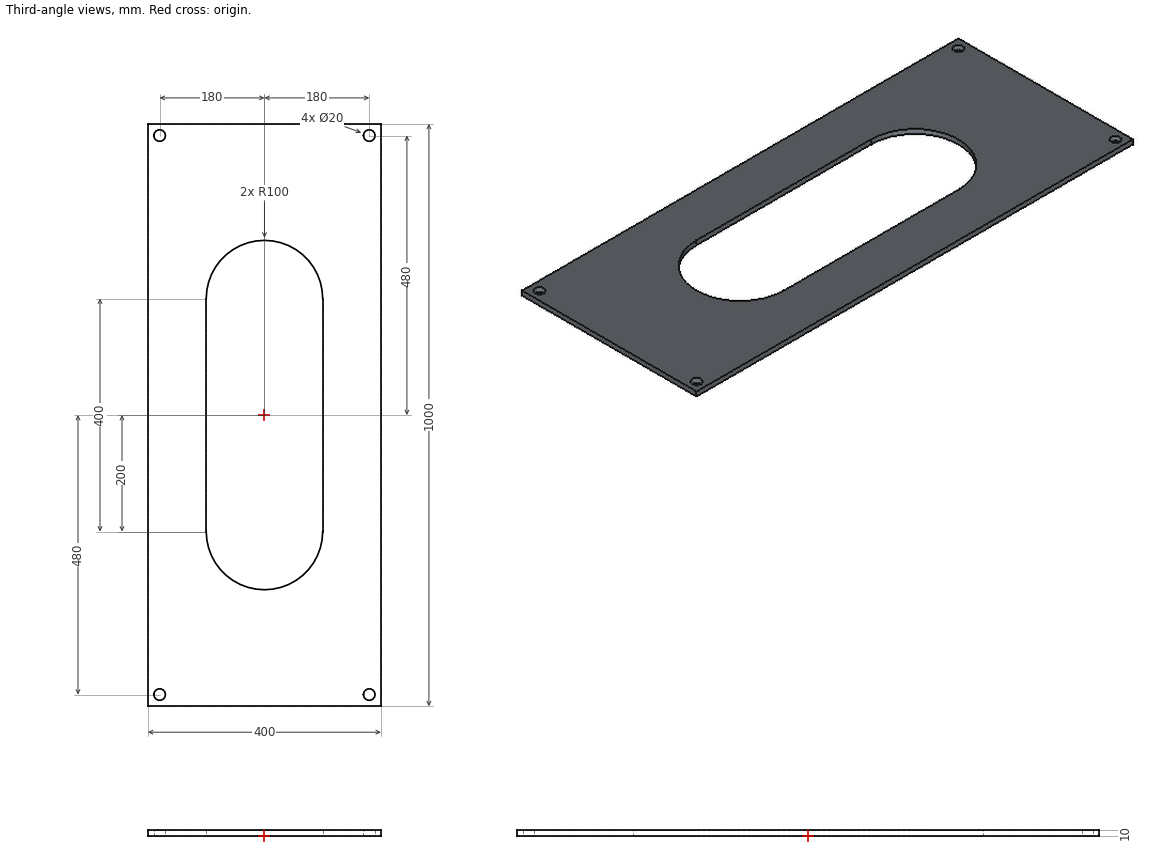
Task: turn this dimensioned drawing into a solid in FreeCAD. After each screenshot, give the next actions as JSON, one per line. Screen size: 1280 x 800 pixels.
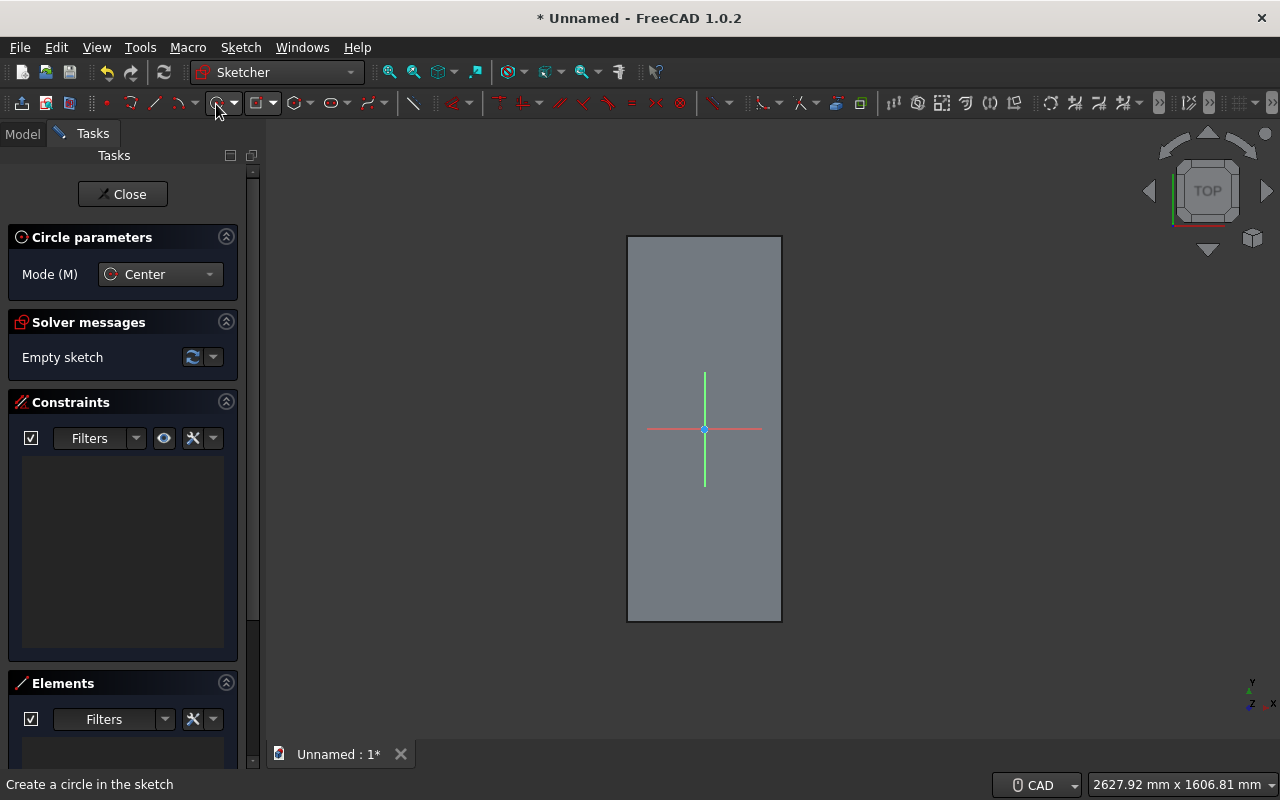
{"action": "scroll", "coordinate": [774, 244], "scroll_direction": "up", "scroll_amount": 9}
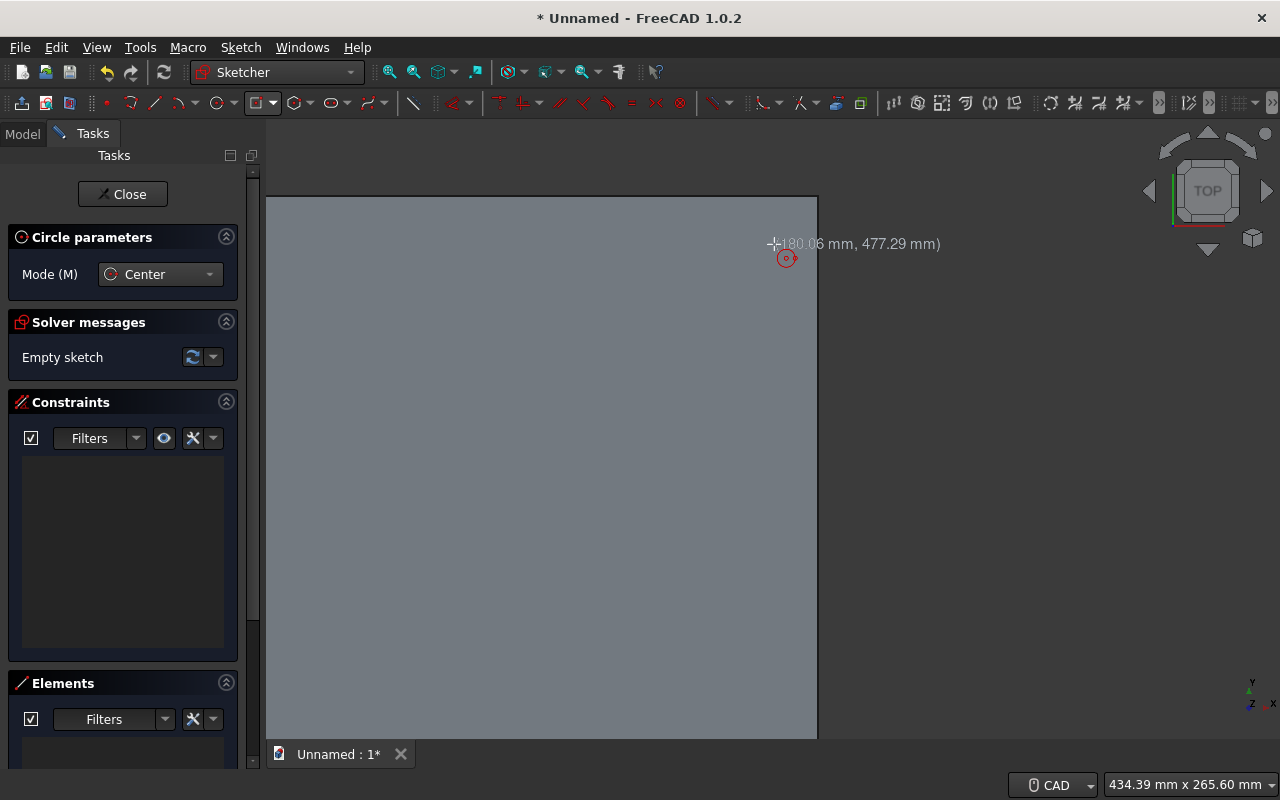
{"action": "scroll", "coordinate": [774, 244], "scroll_direction": "down", "scroll_amount": 9}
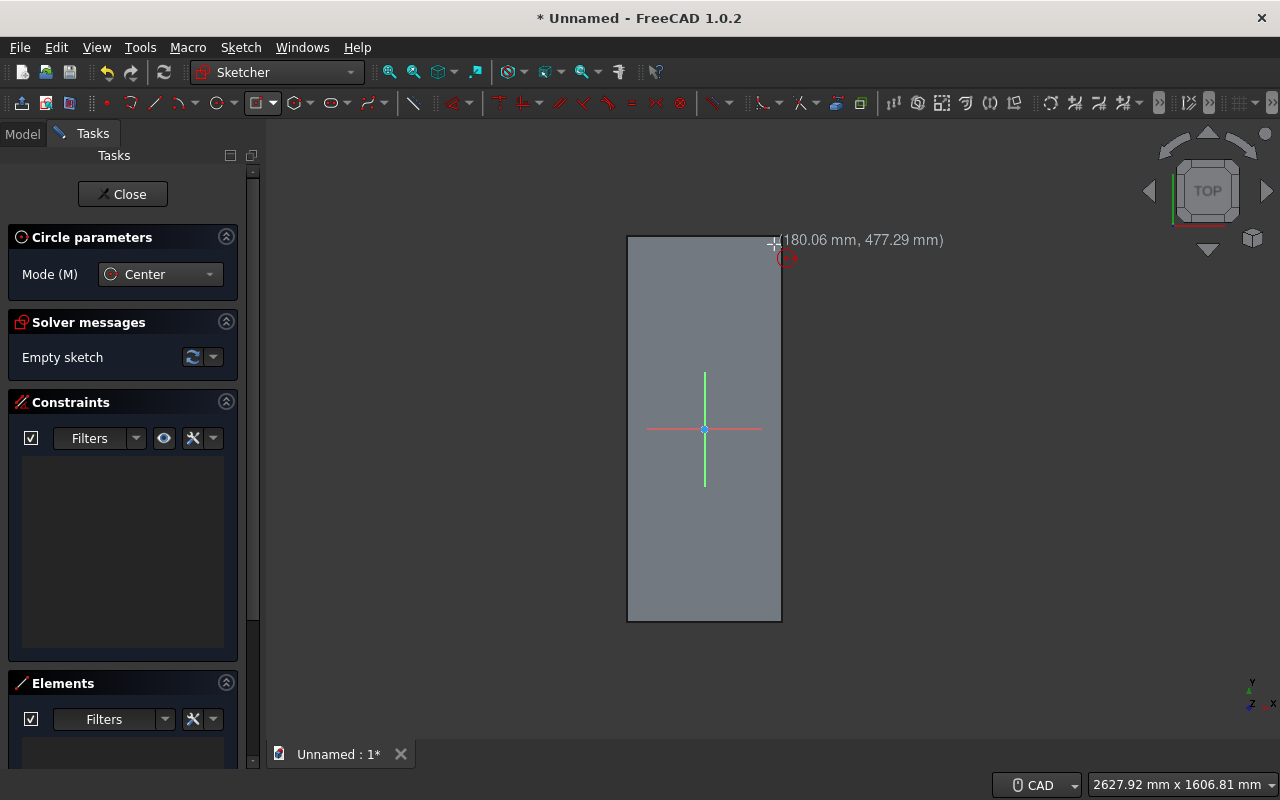
{"action": "left_click", "coordinate": [774, 244]}
{"action": "mouse_move", "coordinate": [777, 241]}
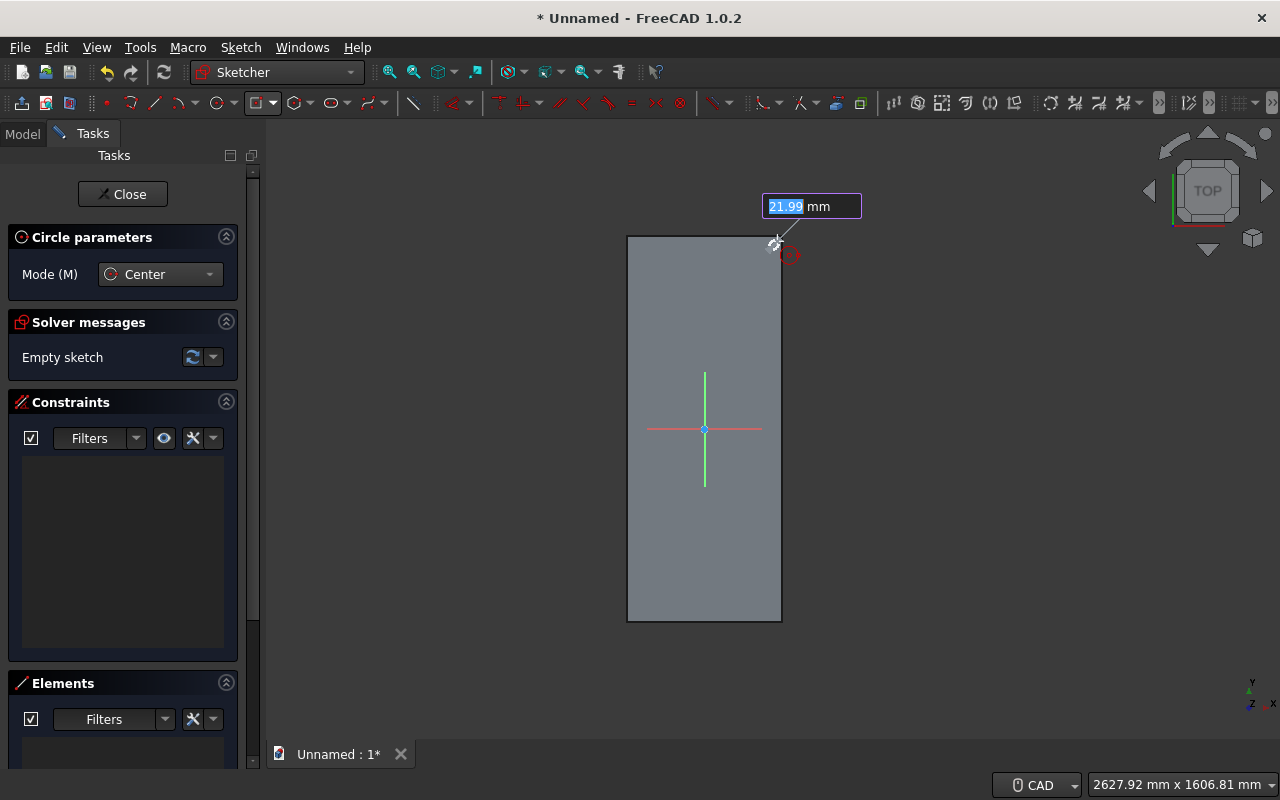
{"action": "type", "text": "20"}
{"action": "key", "text": "Return"}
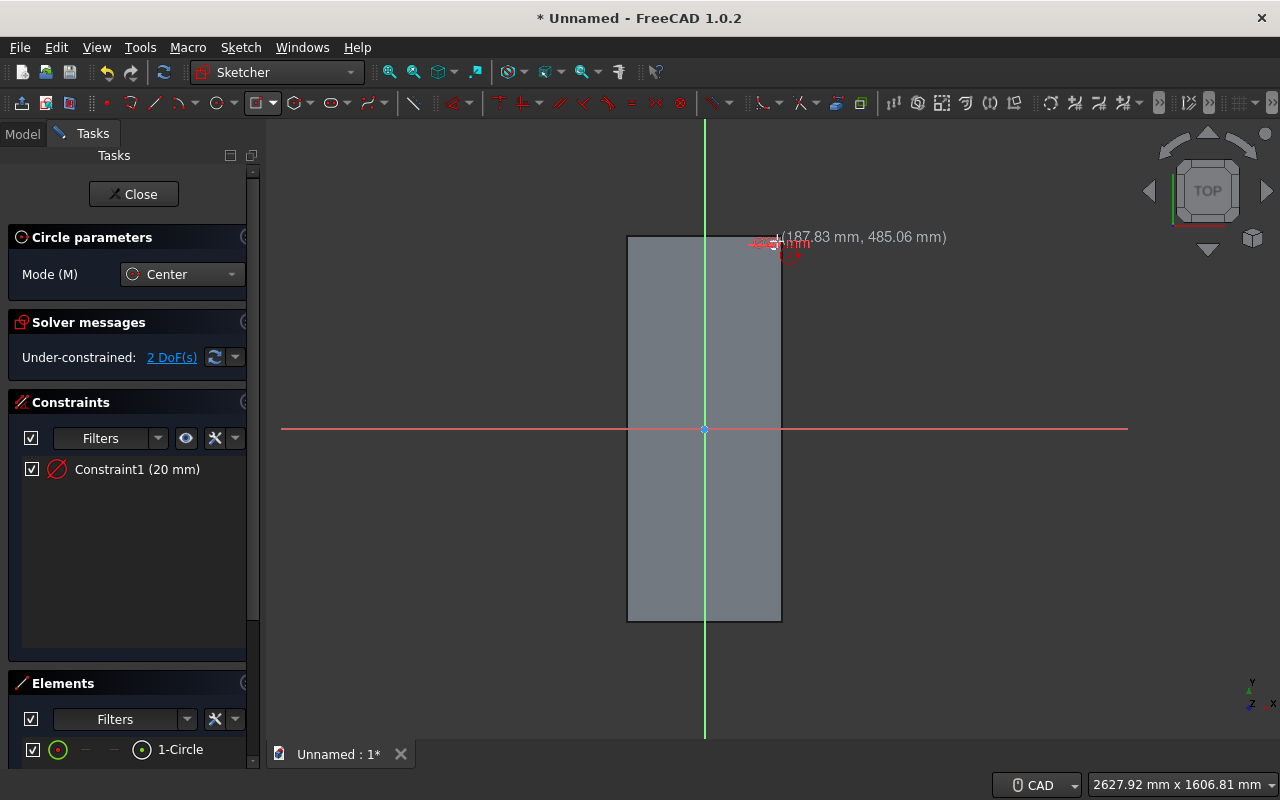
{"action": "scroll", "coordinate": [635, 244], "scroll_direction": "up", "scroll_amount": 9}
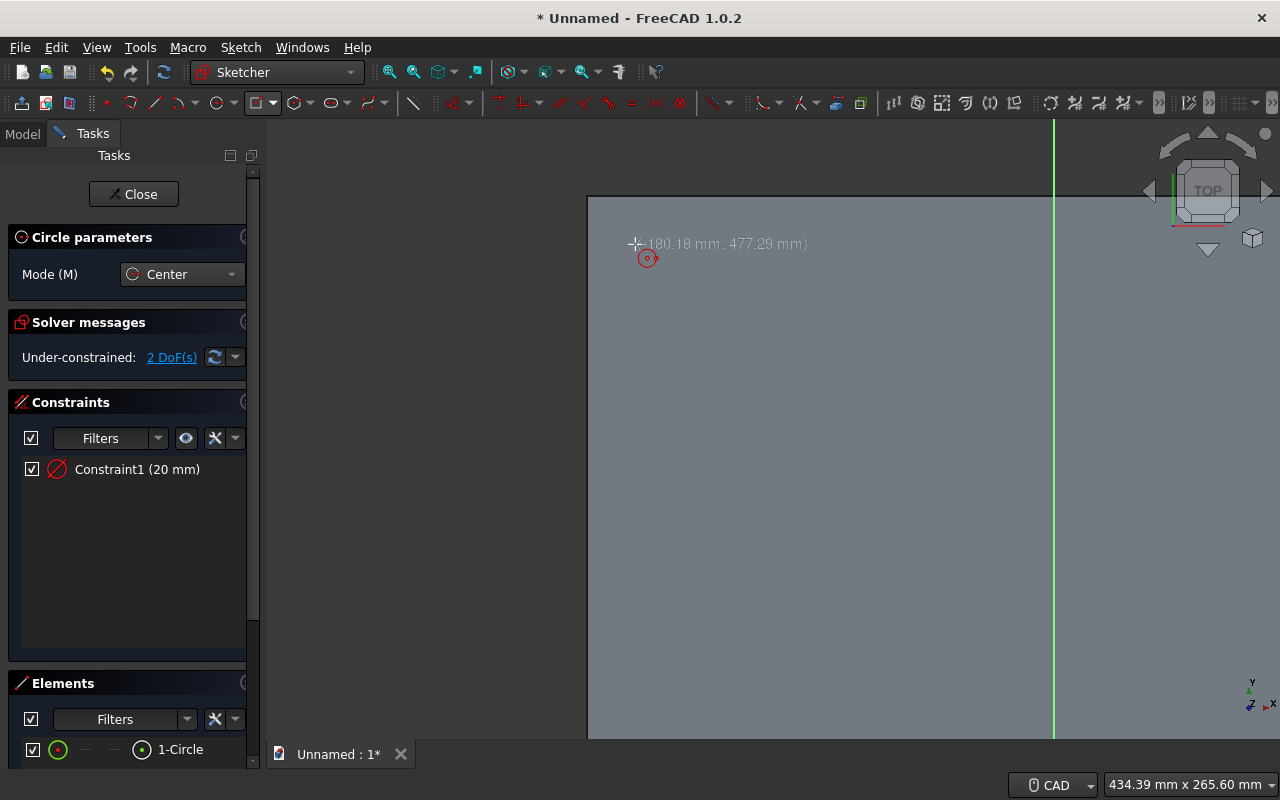
{"action": "scroll", "coordinate": [635, 244], "scroll_direction": "down", "scroll_amount": 9}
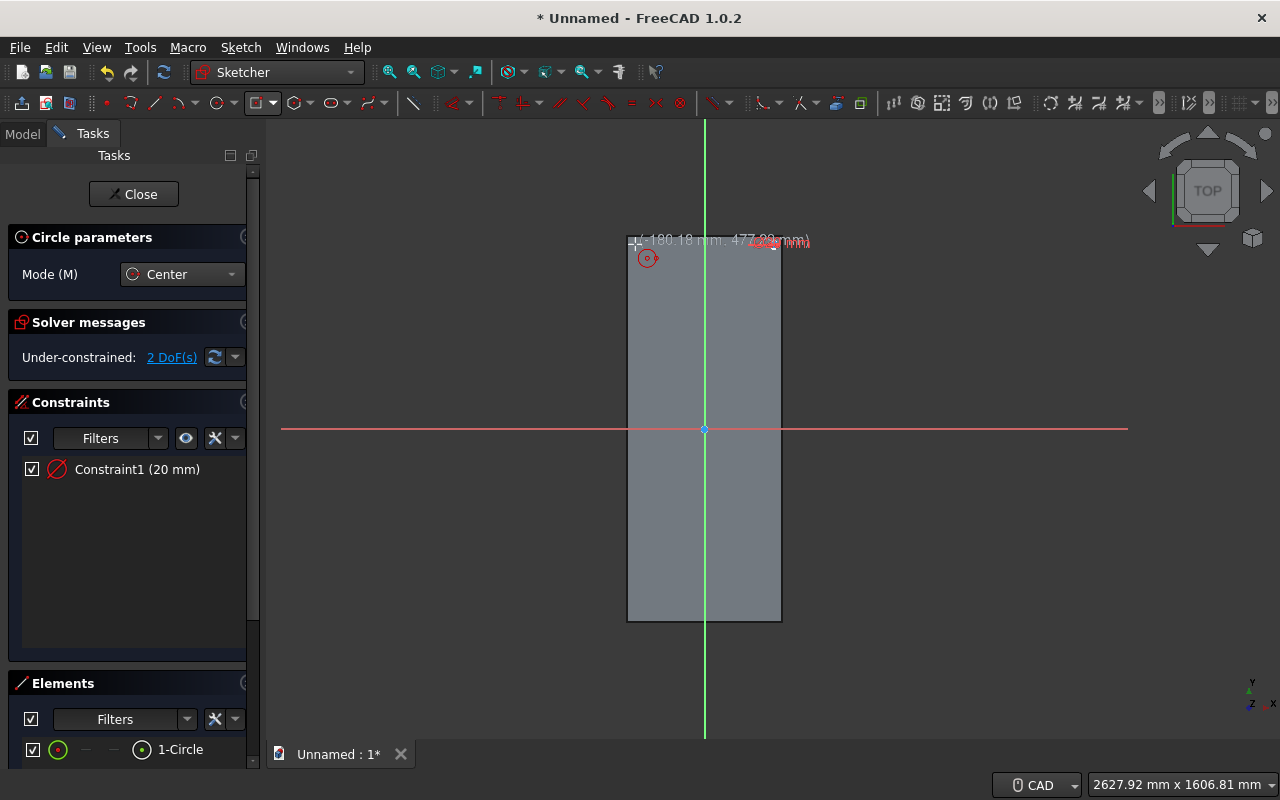
{"action": "left_click", "coordinate": [635, 244]}
{"action": "mouse_move", "coordinate": [638, 241]}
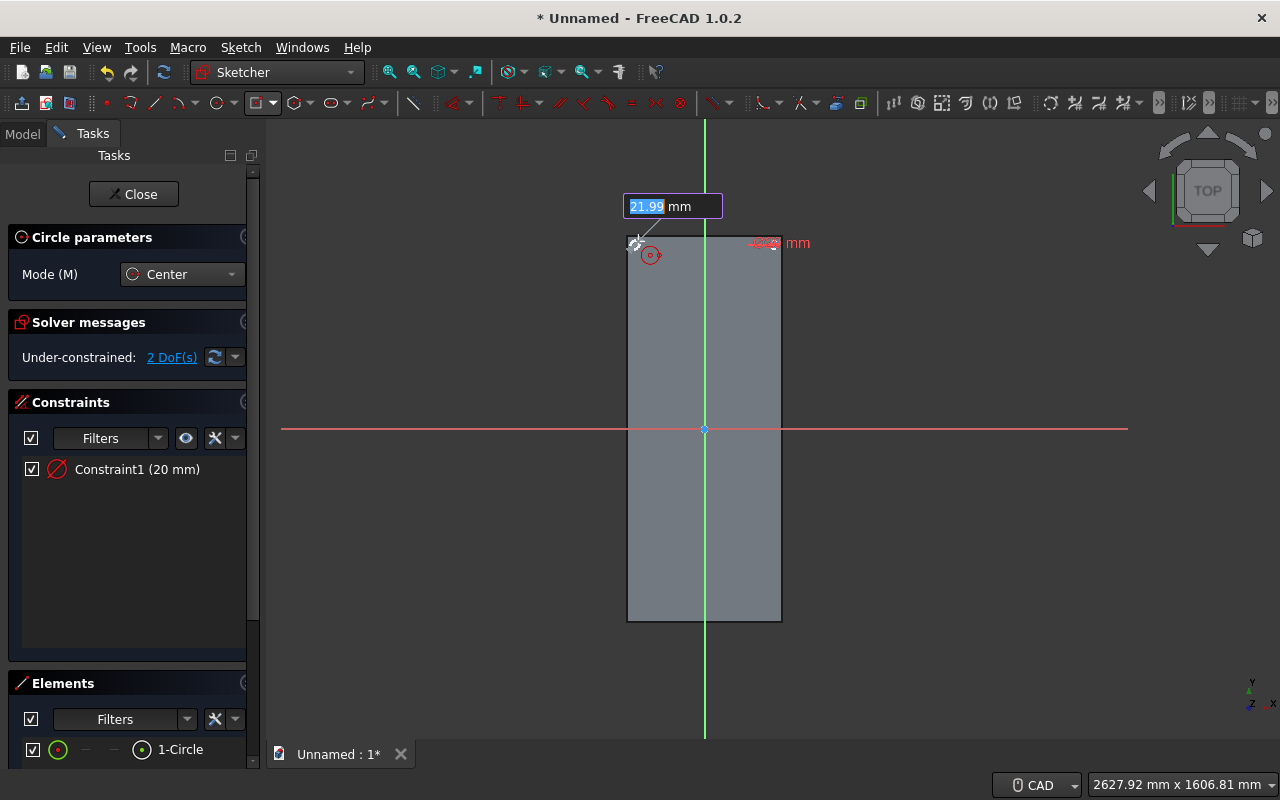
{"action": "type", "text": "20"}
{"action": "key", "text": "Return"}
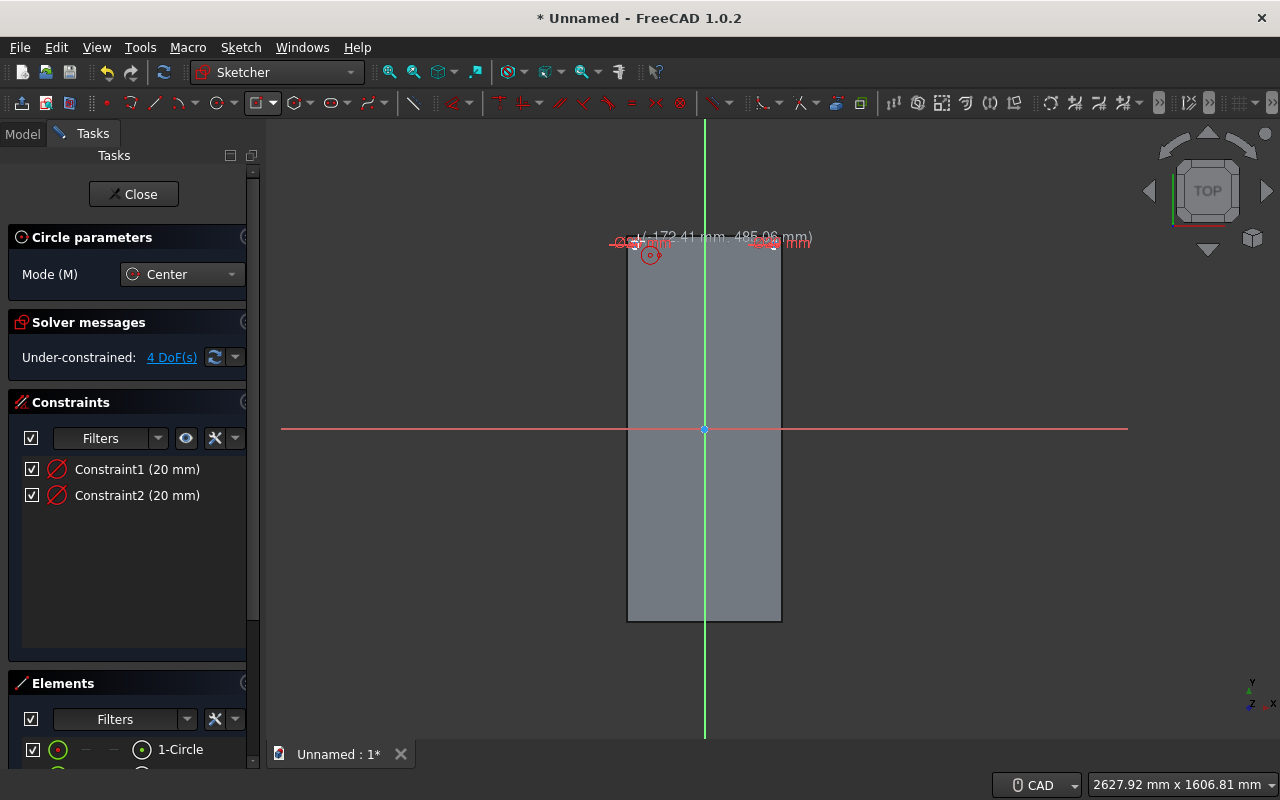
{"action": "scroll", "coordinate": [635, 614], "scroll_direction": "up", "scroll_amount": 9}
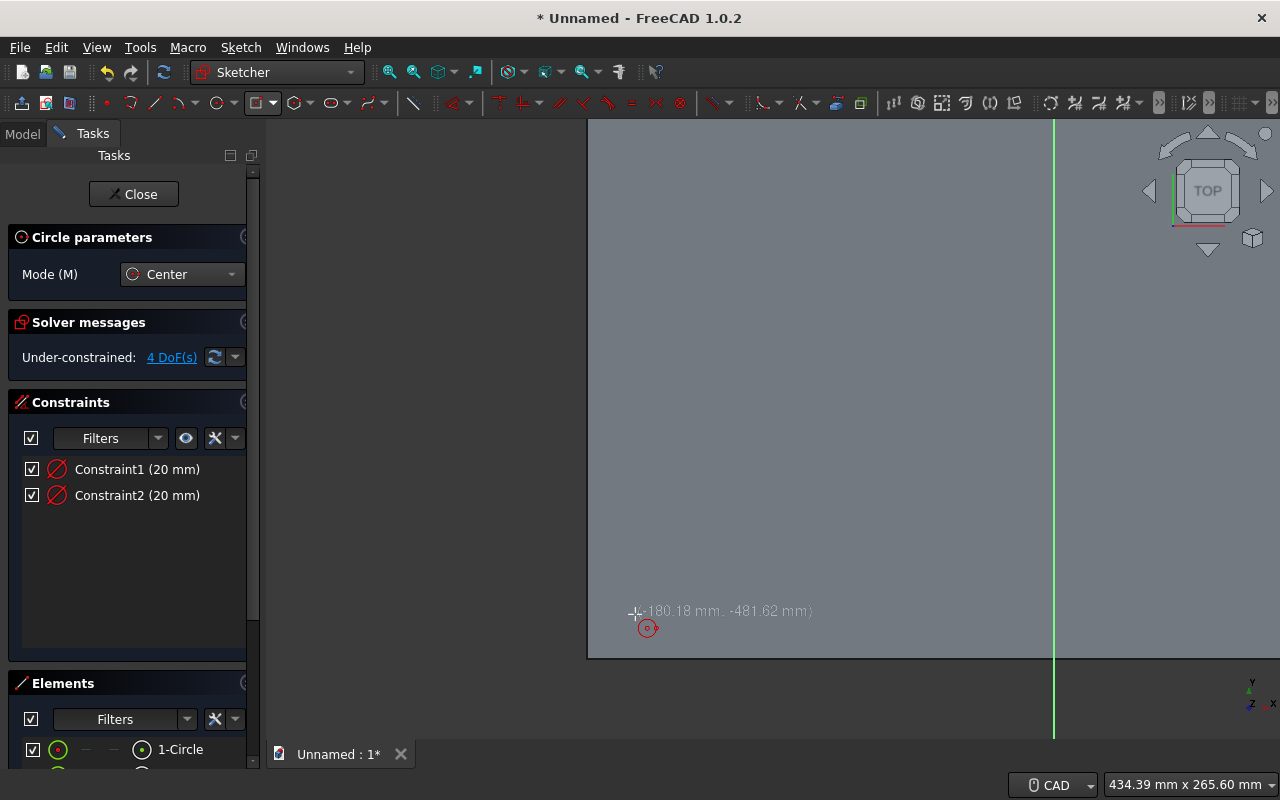
{"action": "scroll", "coordinate": [635, 615], "scroll_direction": "down", "scroll_amount": 9}